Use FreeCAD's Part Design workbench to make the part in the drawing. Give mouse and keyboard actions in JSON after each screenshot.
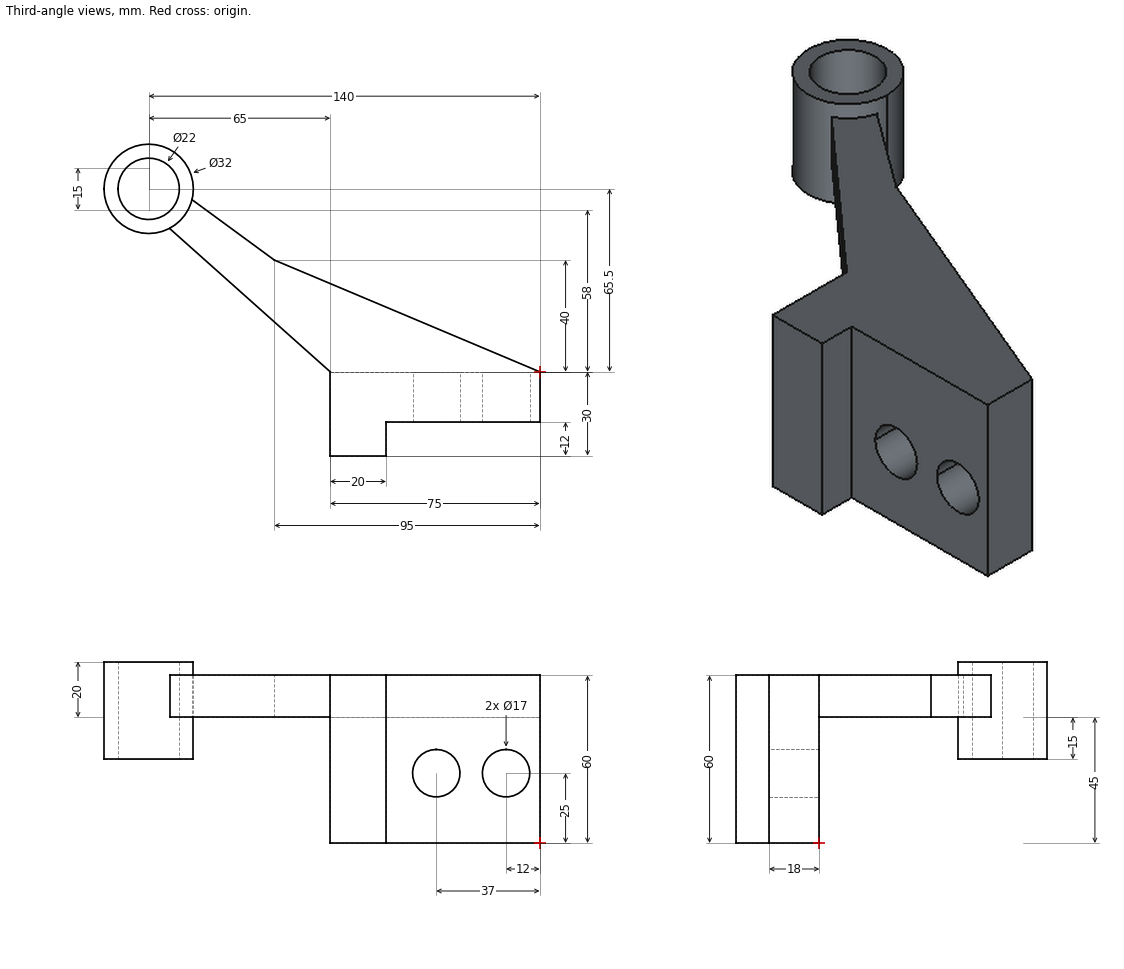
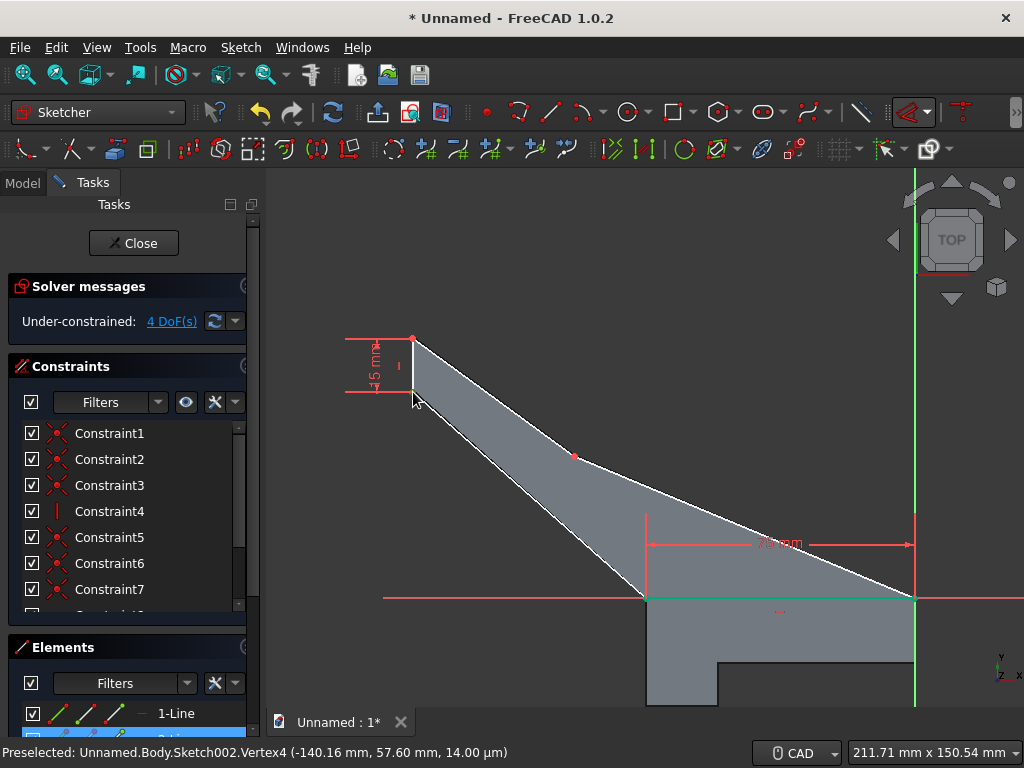
{"action": "key", "text": "i"}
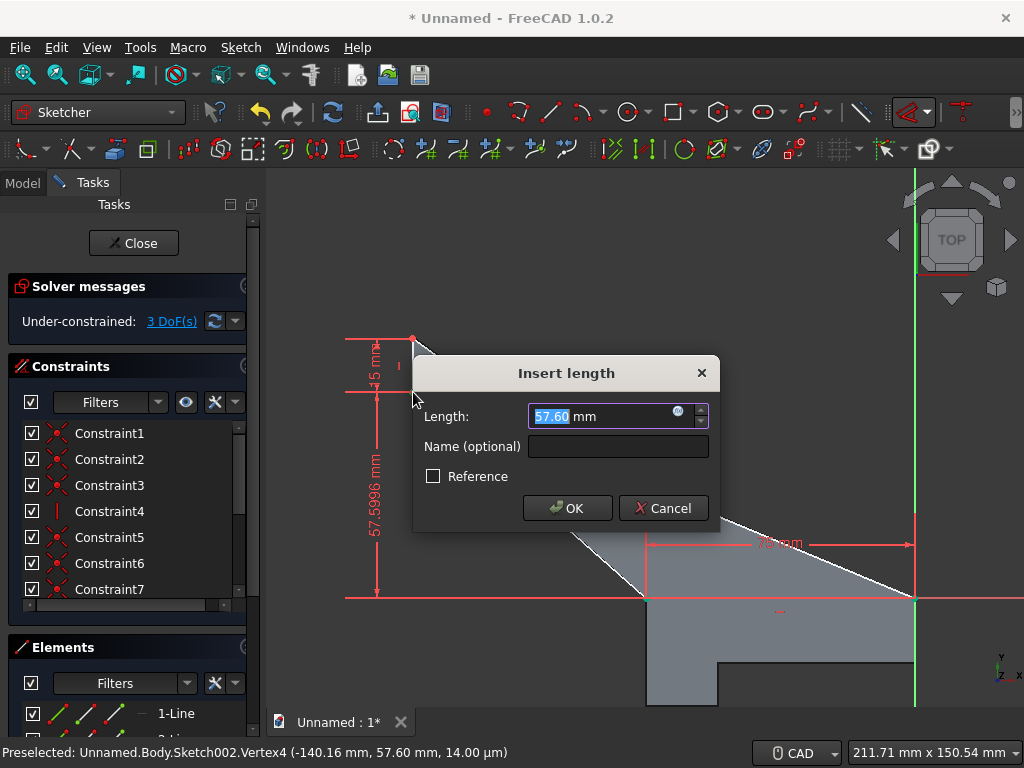
{"action": "type", "text": "58"}
{"action": "key", "text": "Return"}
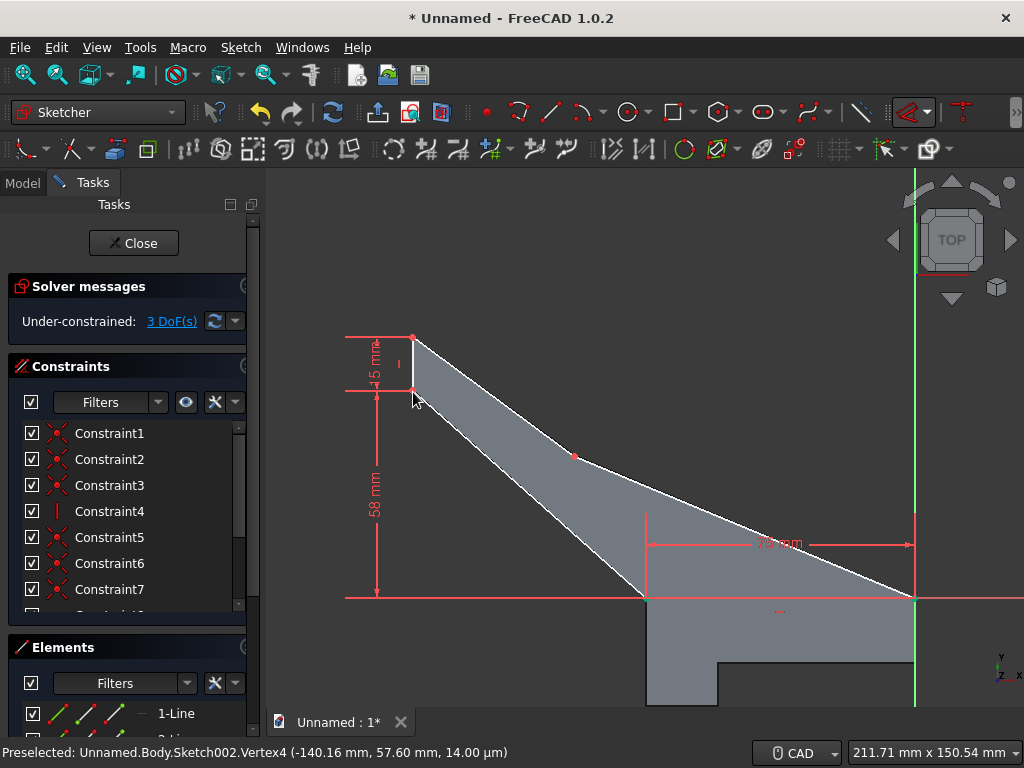
{"action": "left_click", "coordinate": [574, 456]}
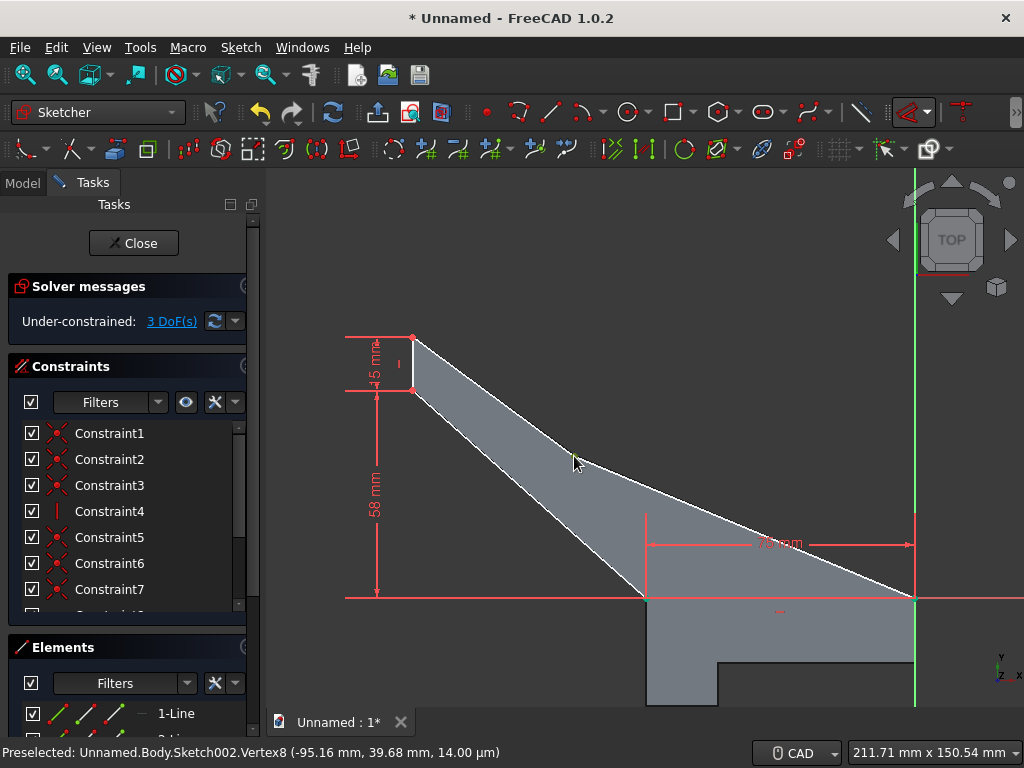
{"action": "key", "text": "l"}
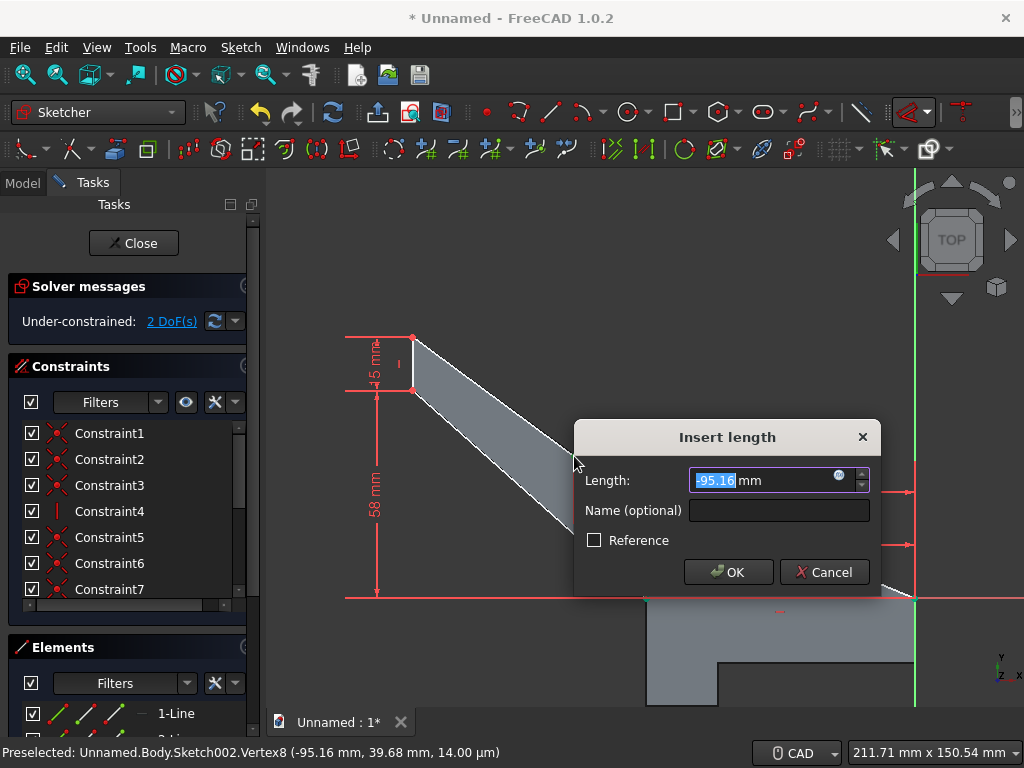
{"action": "type", "text": "-95"}
{"action": "key", "text": "Return"}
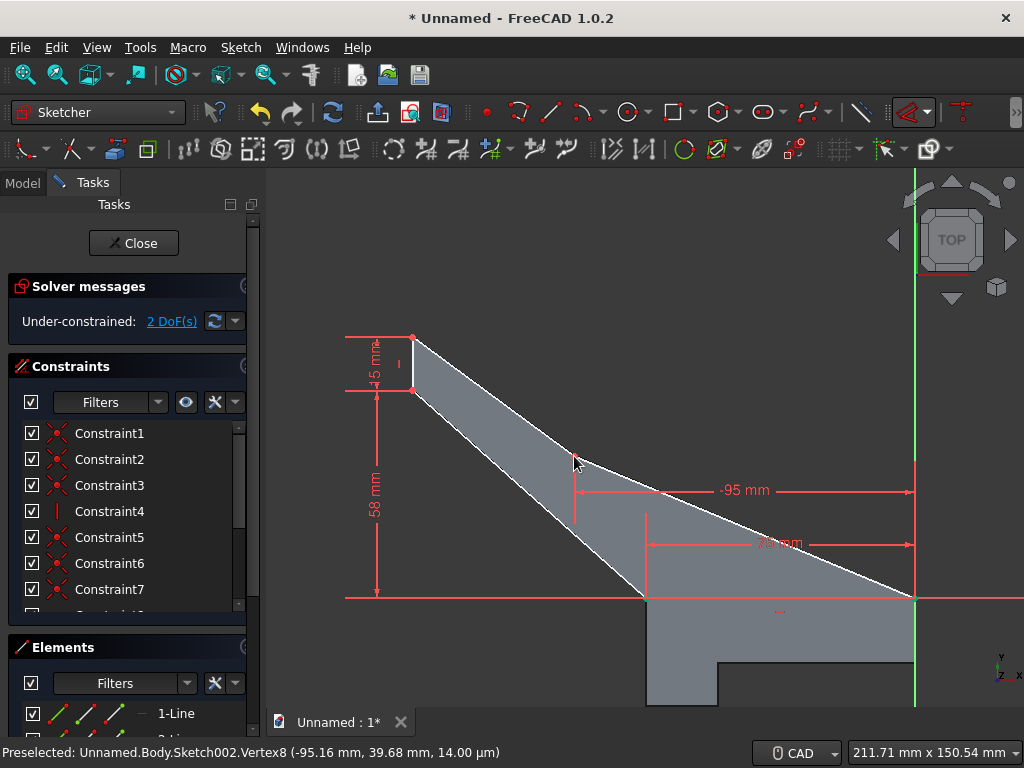
{"action": "left_click", "coordinate": [575, 456]}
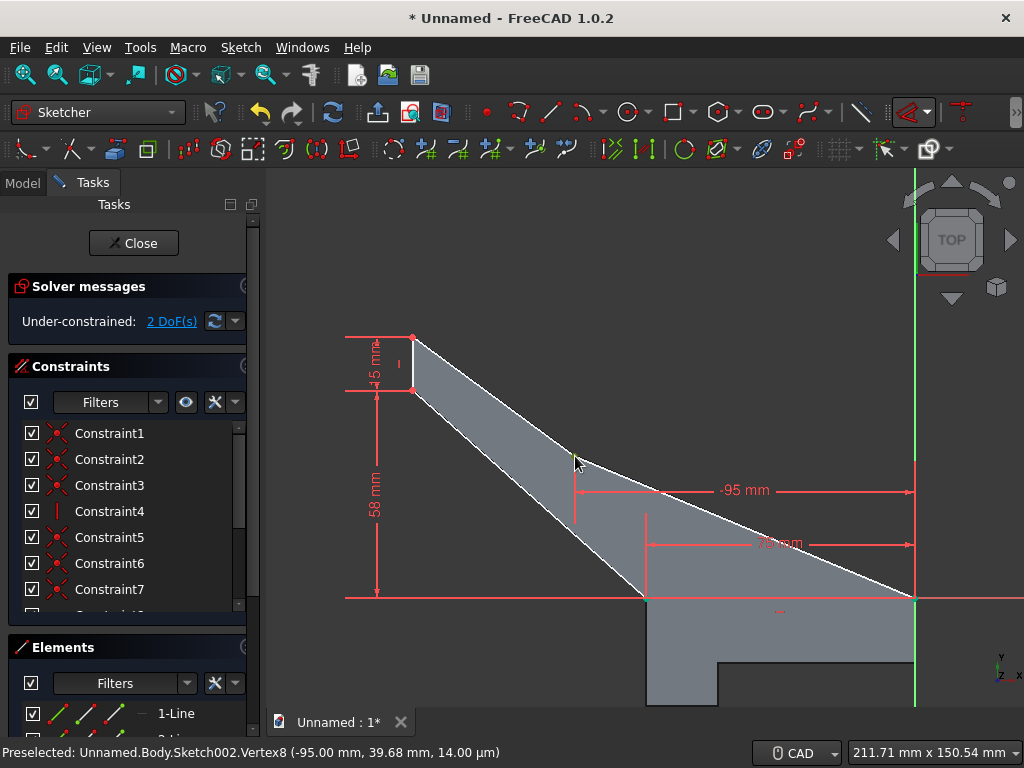
{"action": "left_click", "coordinate": [930, 112]}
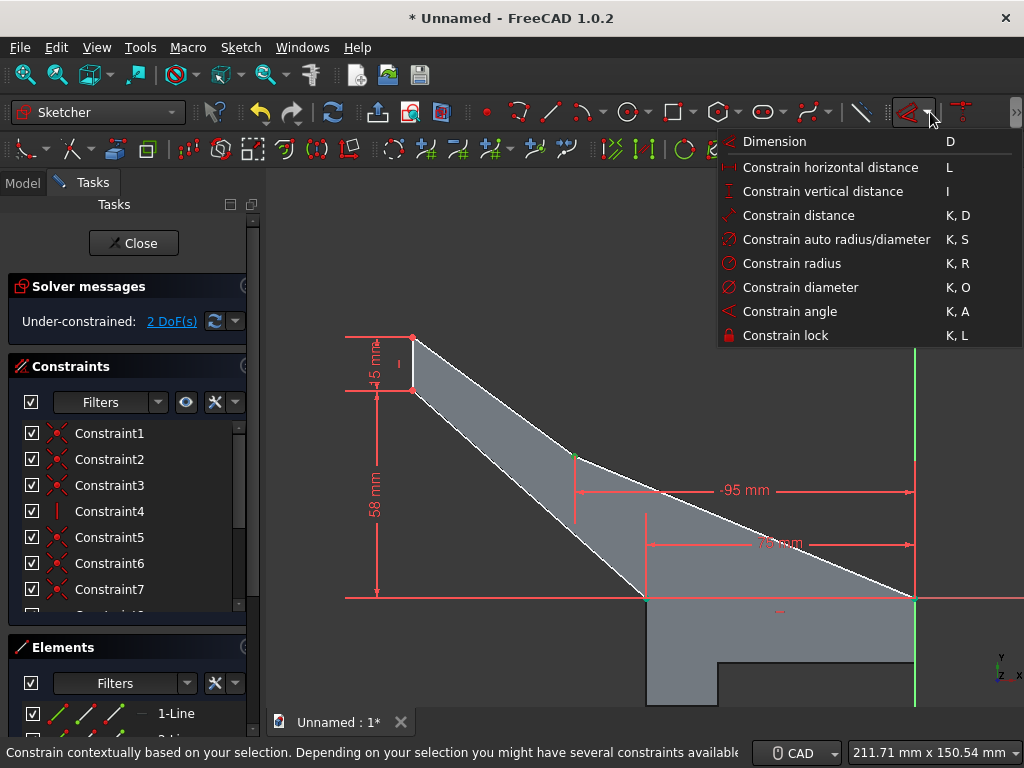
{"action": "left_click", "coordinate": [870, 191]}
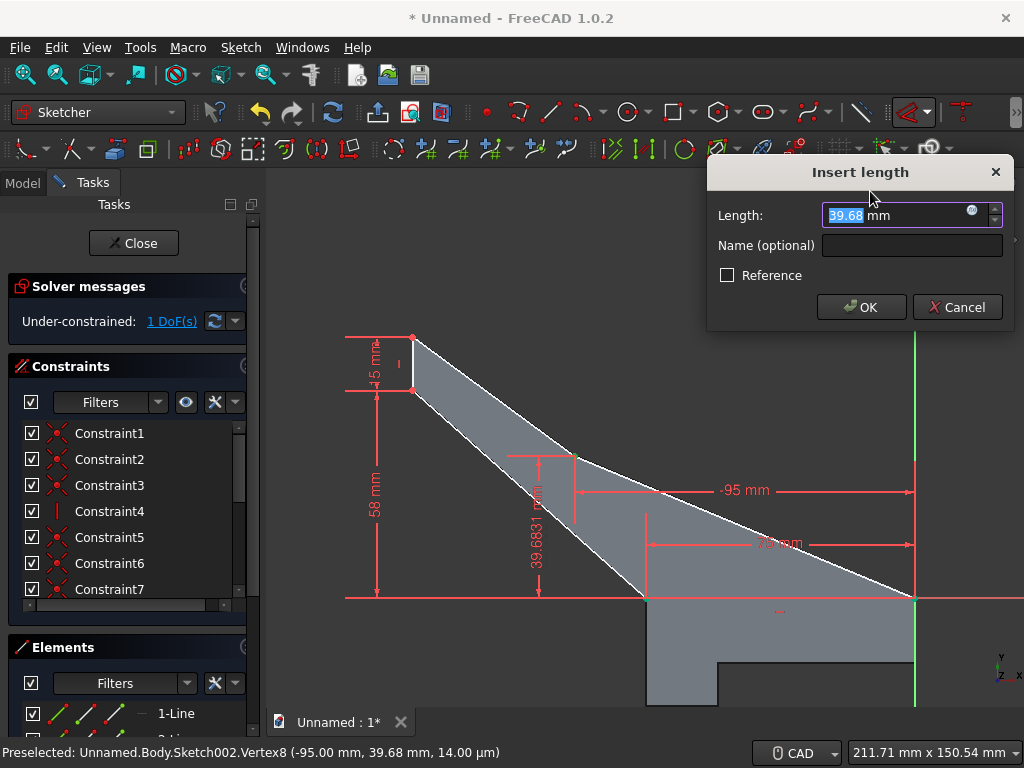
{"action": "type", "text": "40"}
{"action": "key", "text": "Return"}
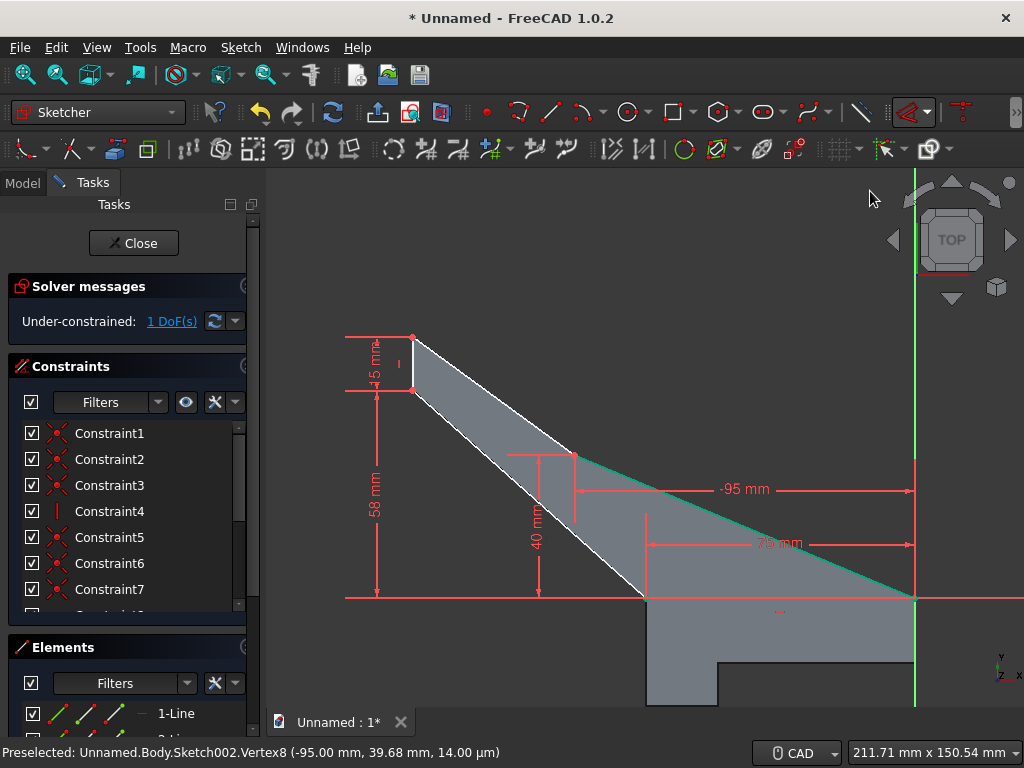
{"action": "left_click", "coordinate": [576, 536]}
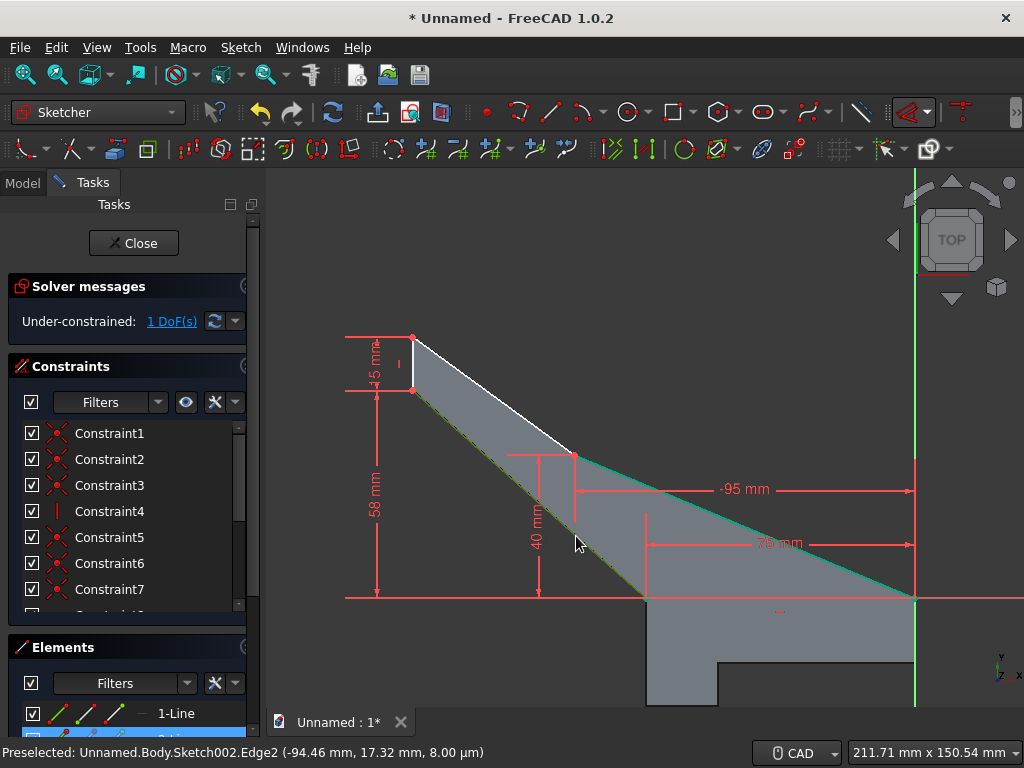
{"action": "key", "text": "l"}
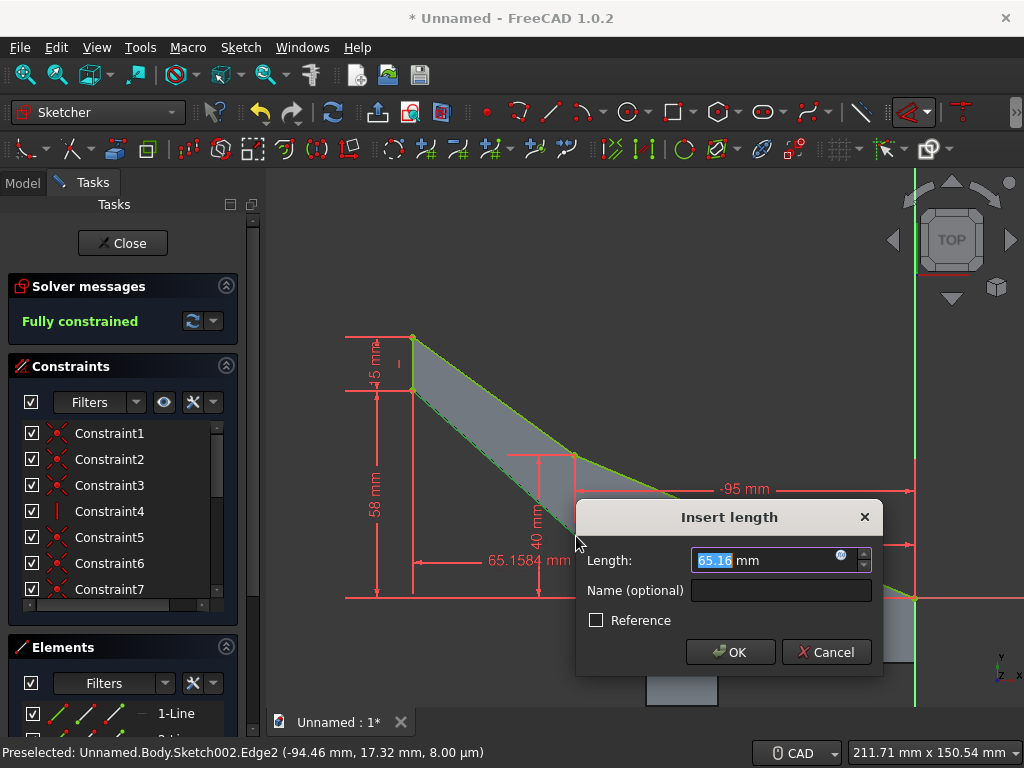
{"action": "type", "text": "65"}
{"action": "key", "text": "Return"}